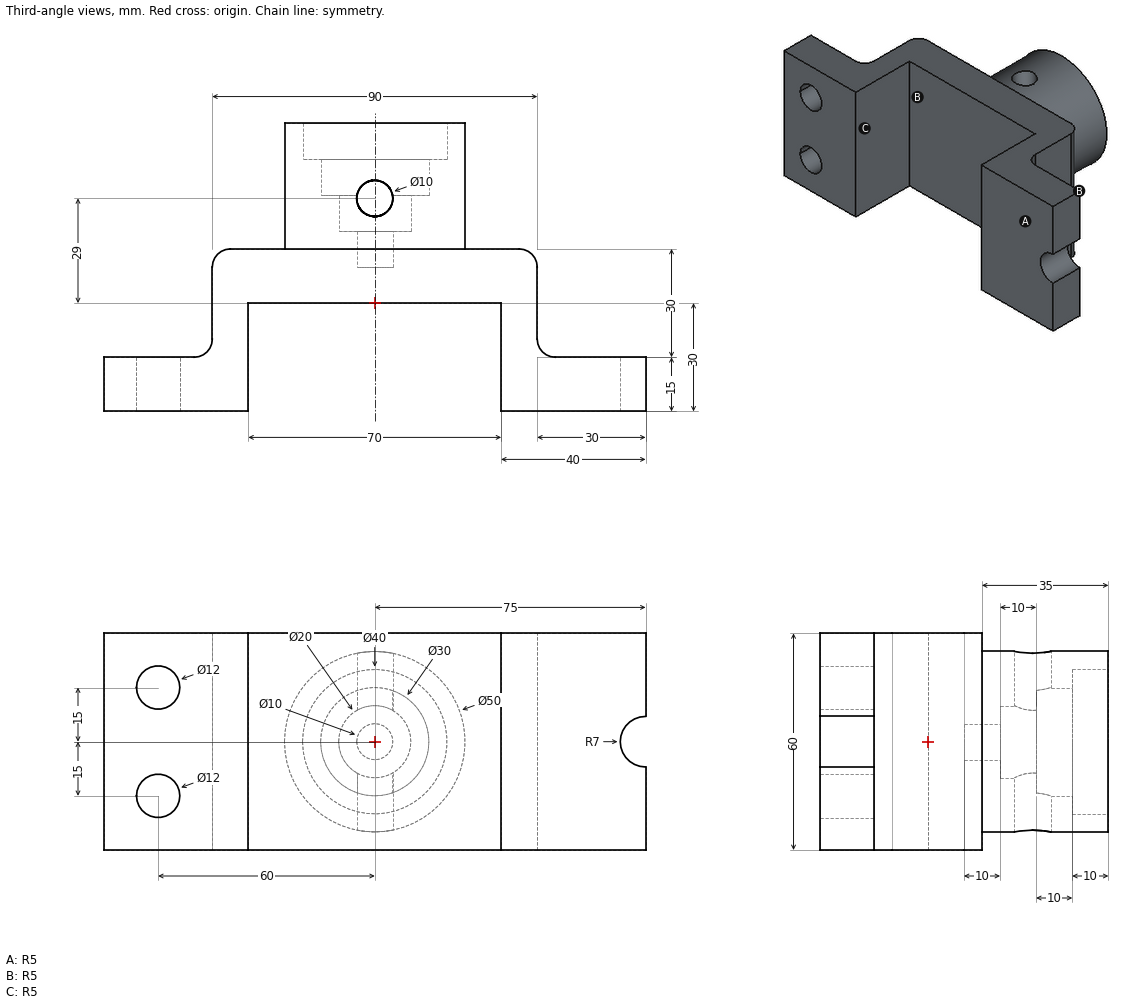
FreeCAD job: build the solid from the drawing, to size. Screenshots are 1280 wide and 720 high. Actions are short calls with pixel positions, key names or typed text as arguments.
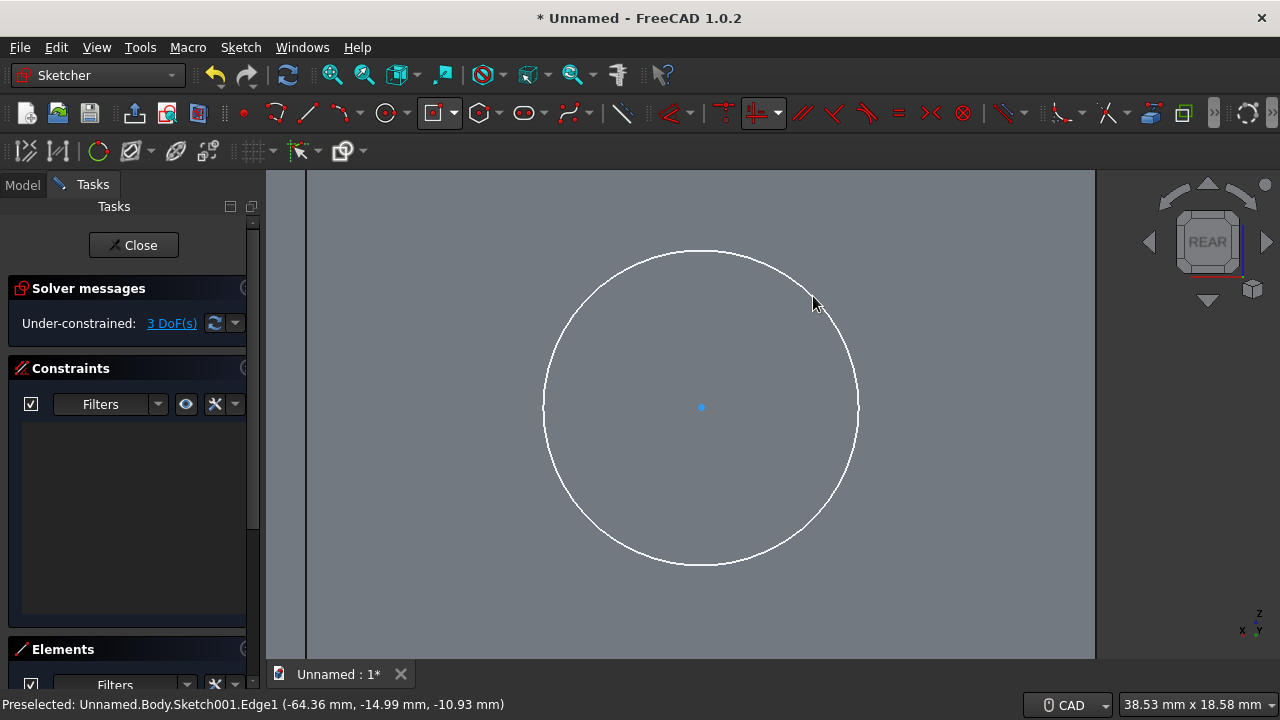
key(d)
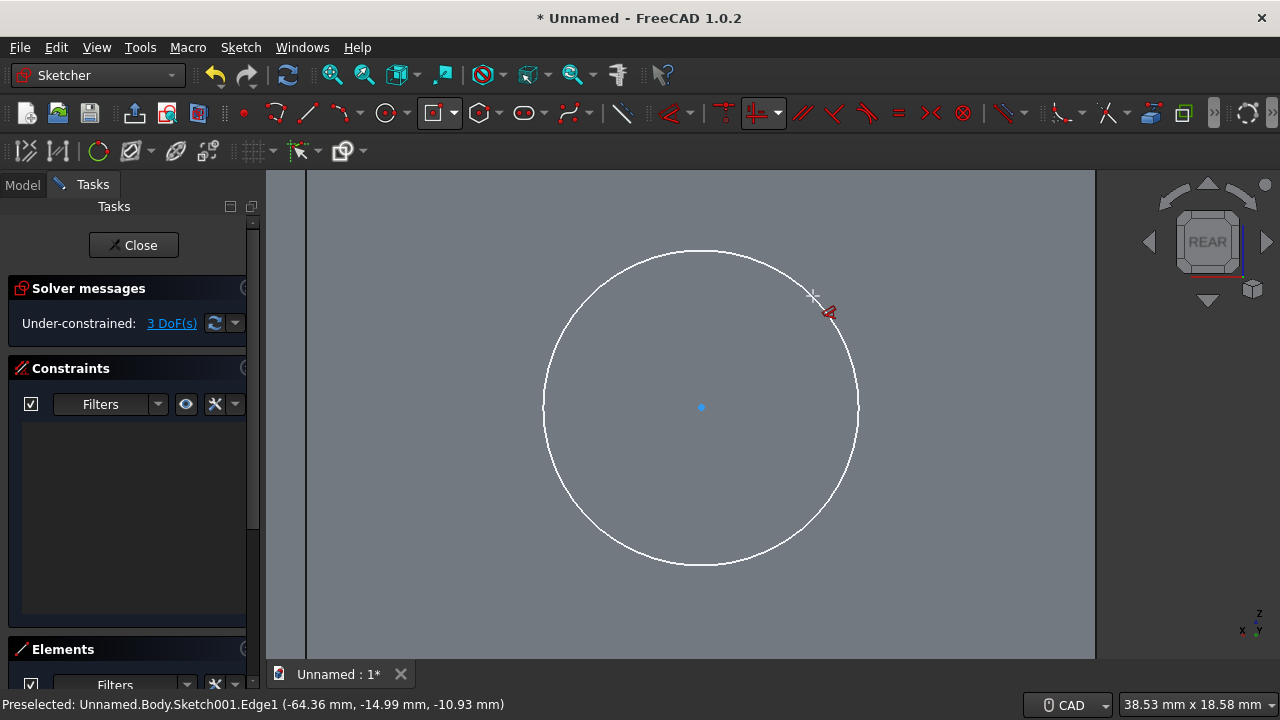
click(812, 296)
click(835, 273)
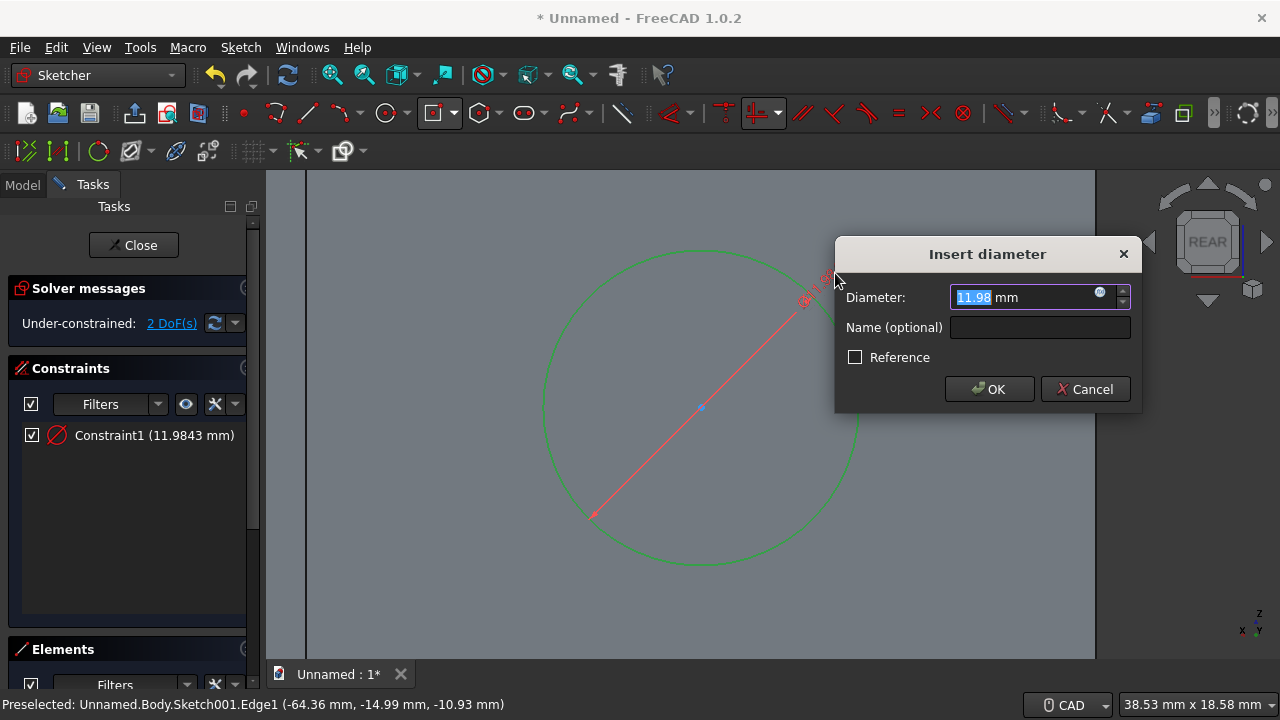
text(12)
key(Return)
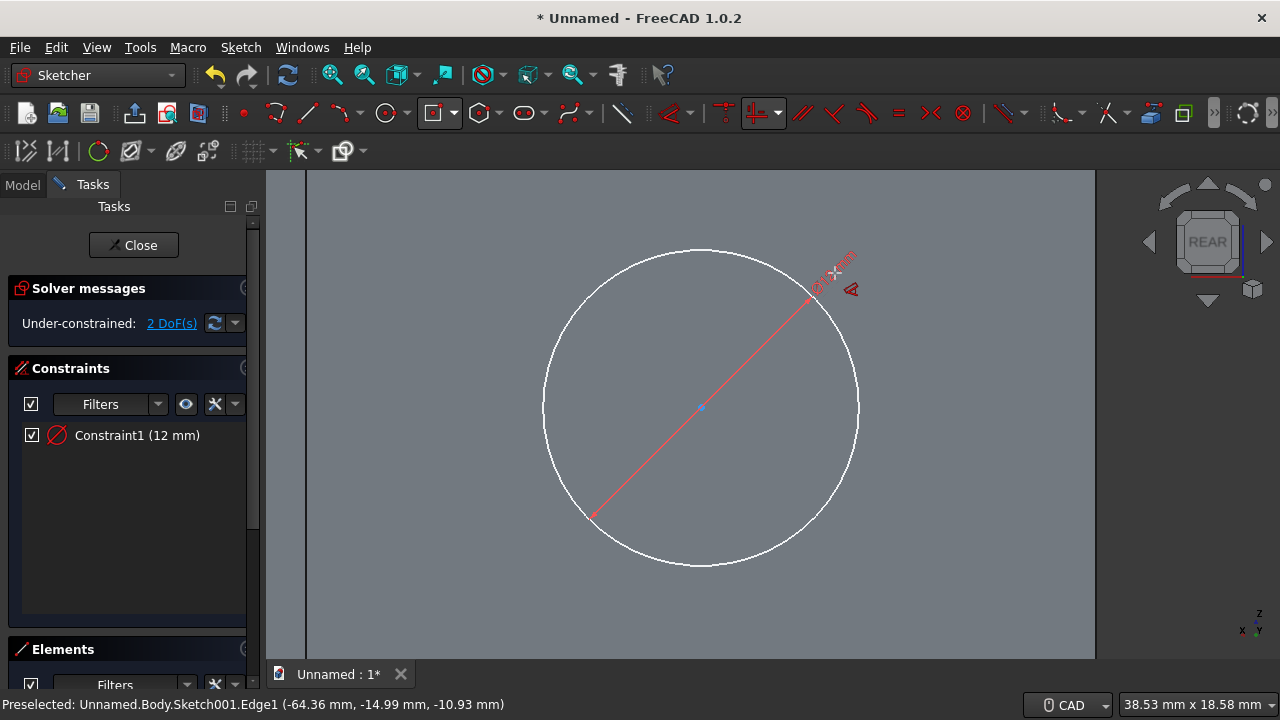
click(701, 408)
click(497, 442)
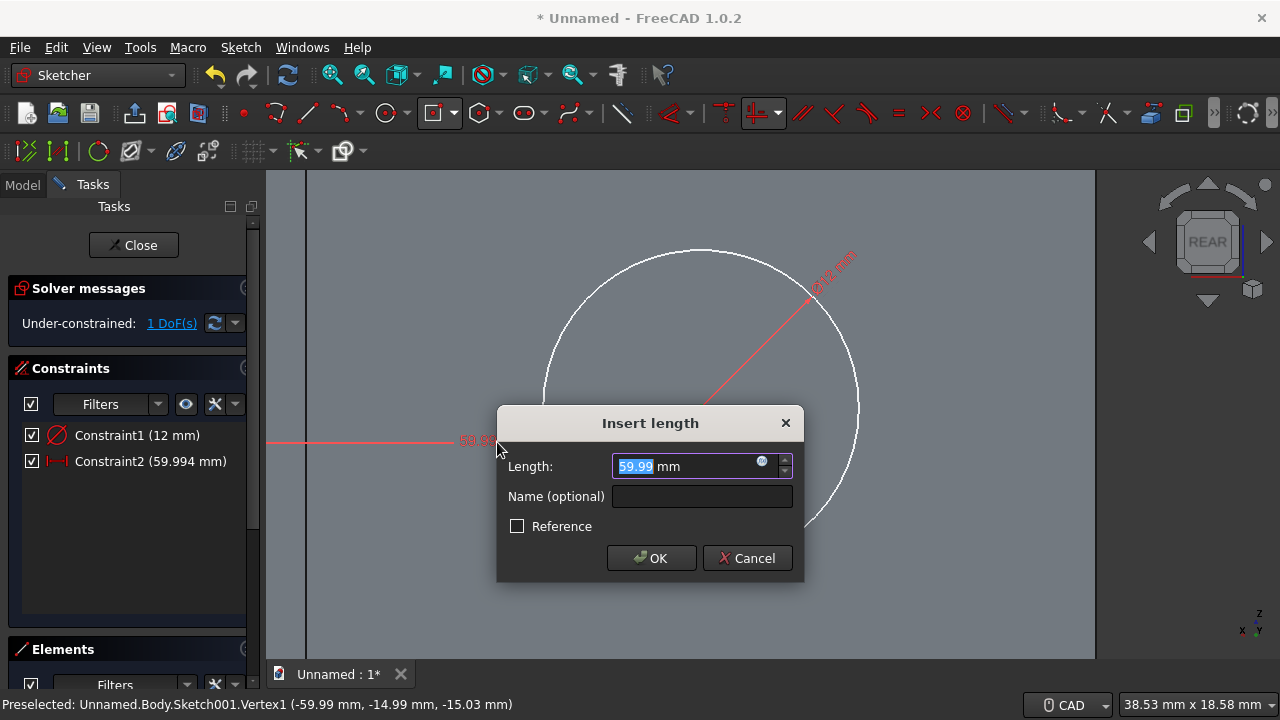
text(60)
key(Return)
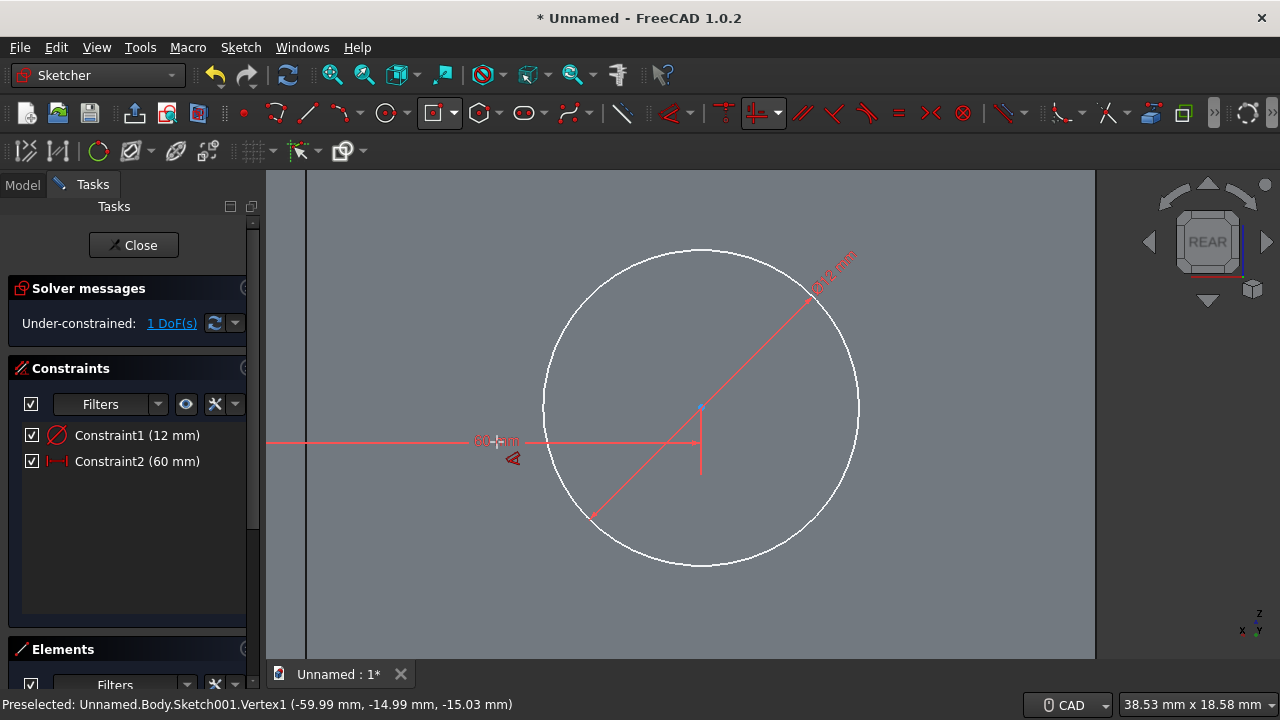
click(701, 408)
click(735, 303)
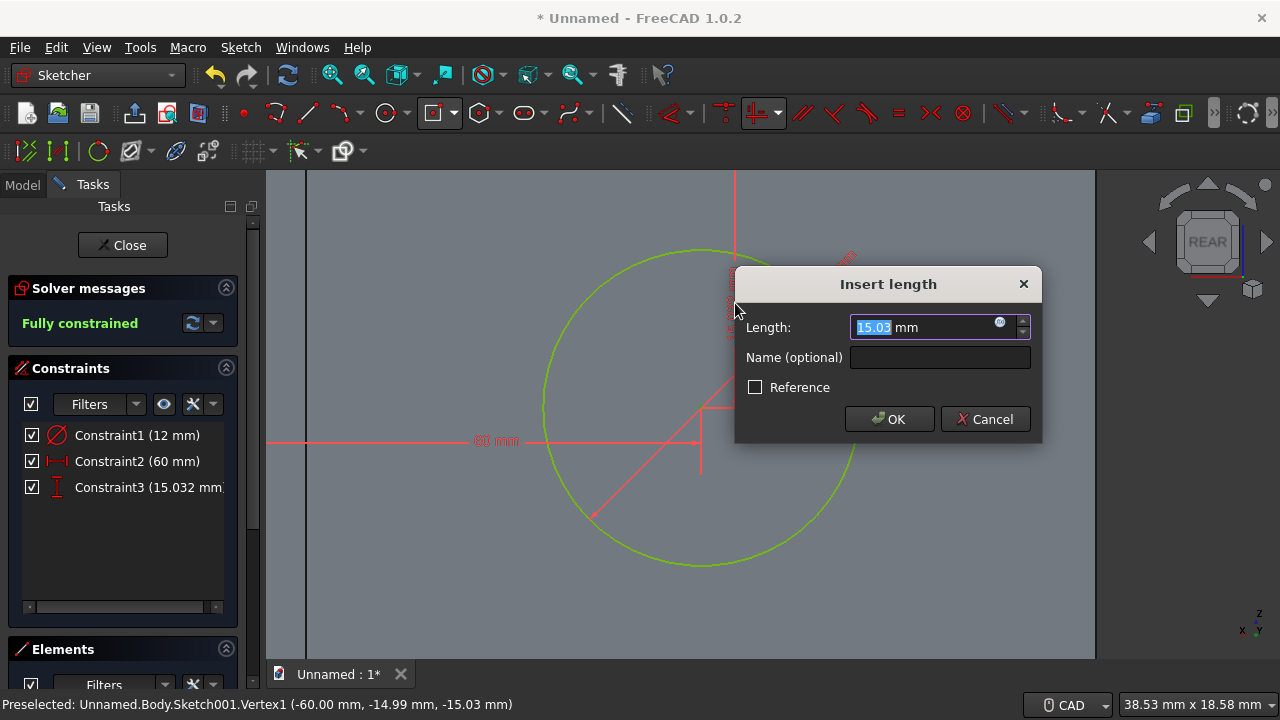
text(15)
key(Return)
key(Escape)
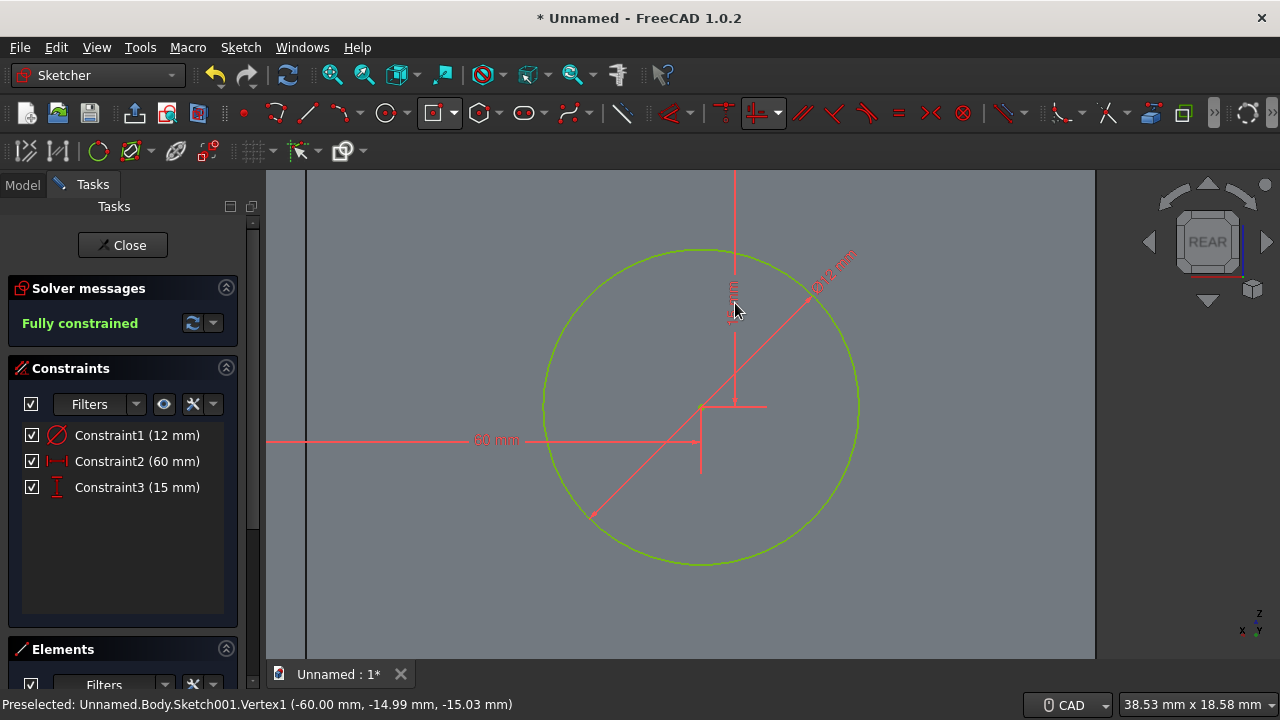
click(123, 245)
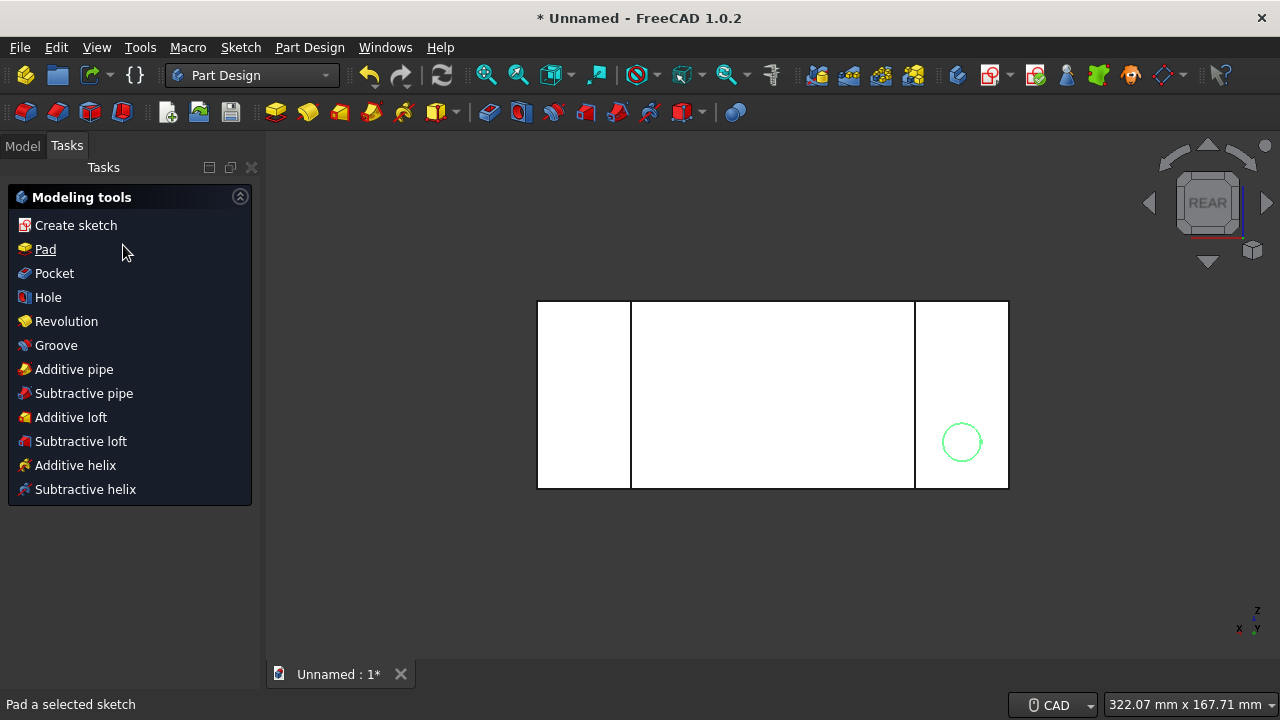
click(490, 112)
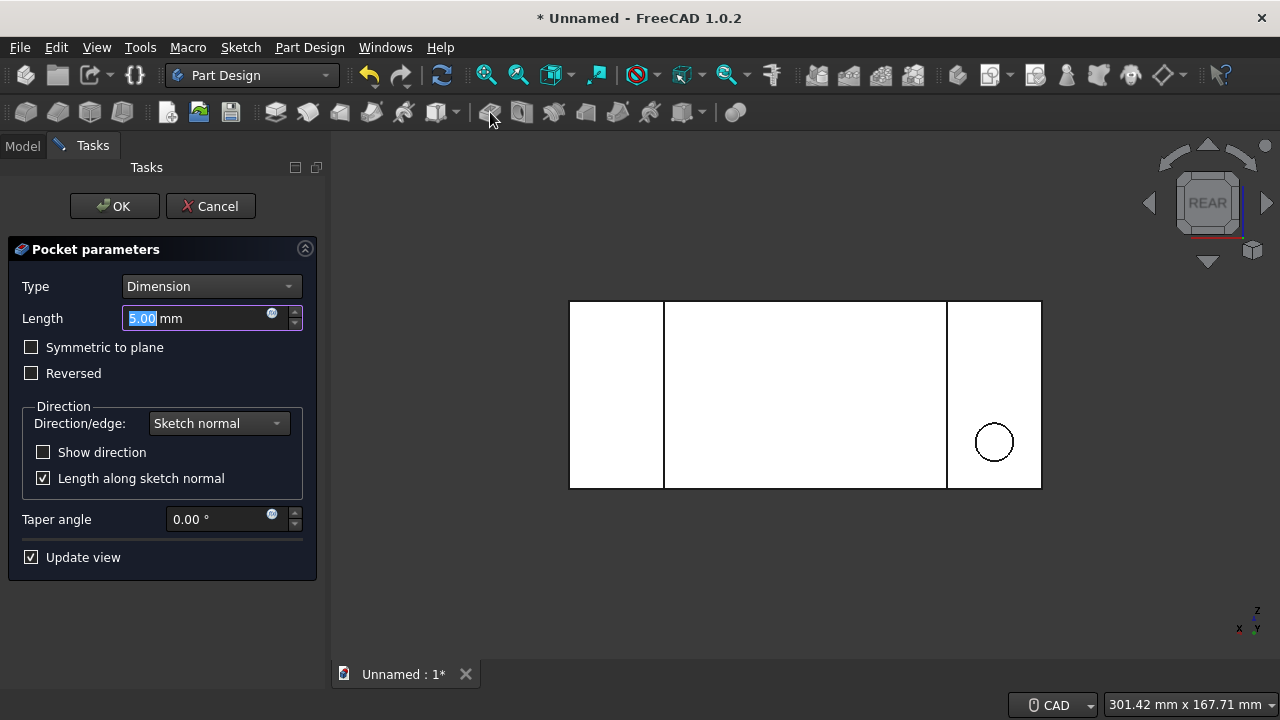
click(212, 286)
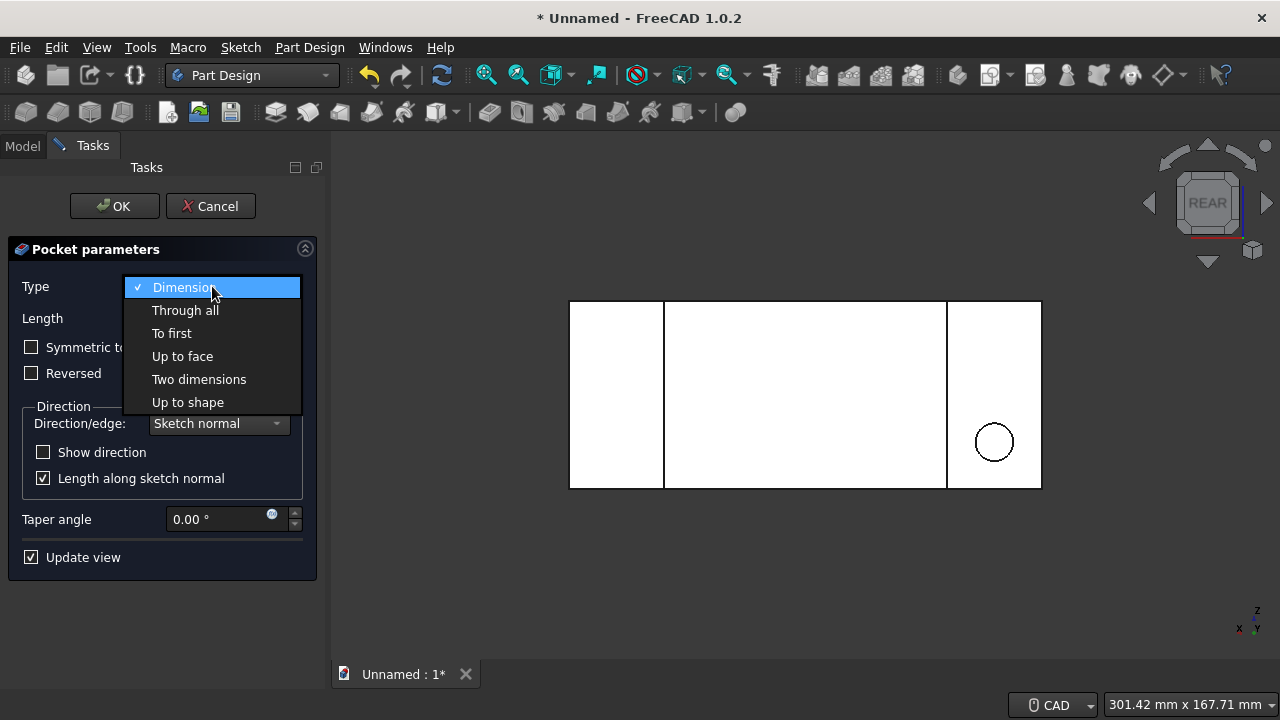
click(212, 334)